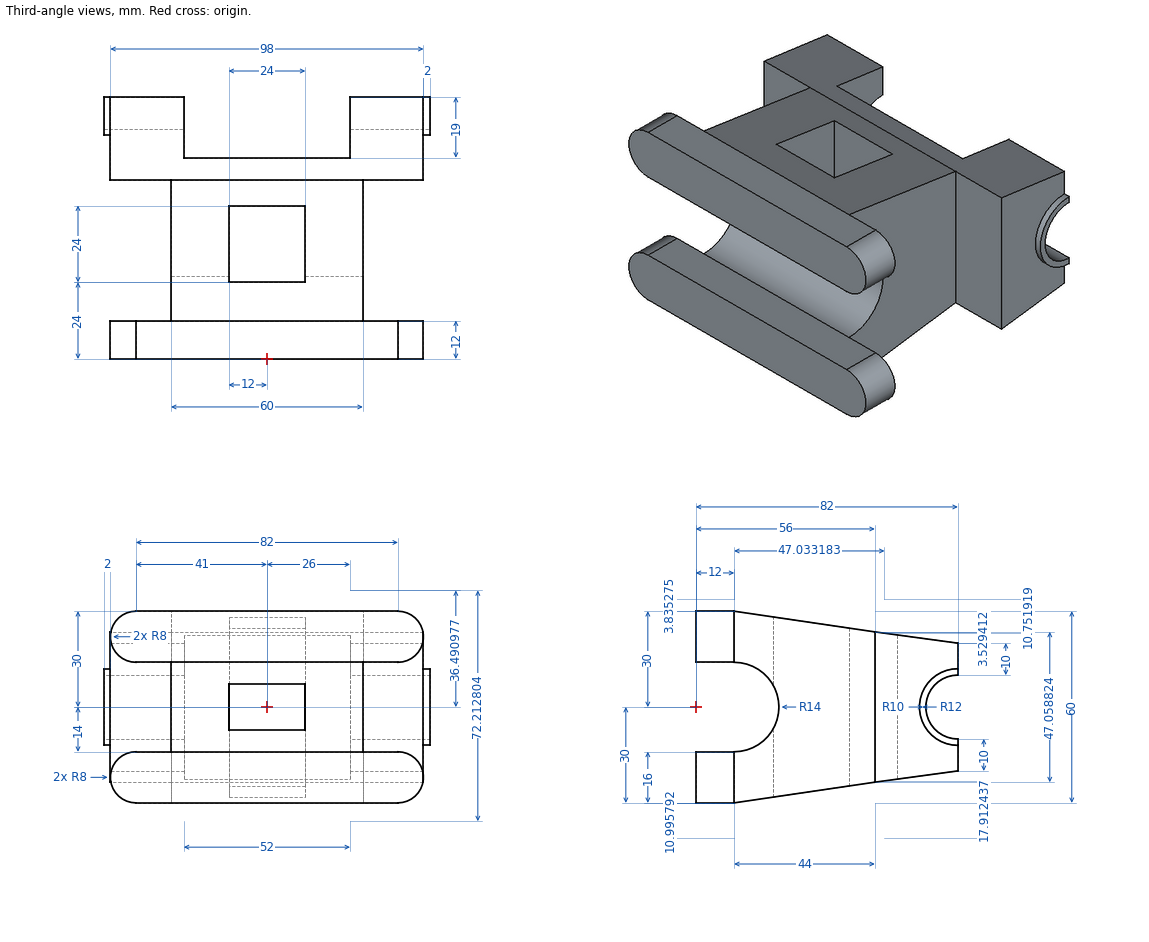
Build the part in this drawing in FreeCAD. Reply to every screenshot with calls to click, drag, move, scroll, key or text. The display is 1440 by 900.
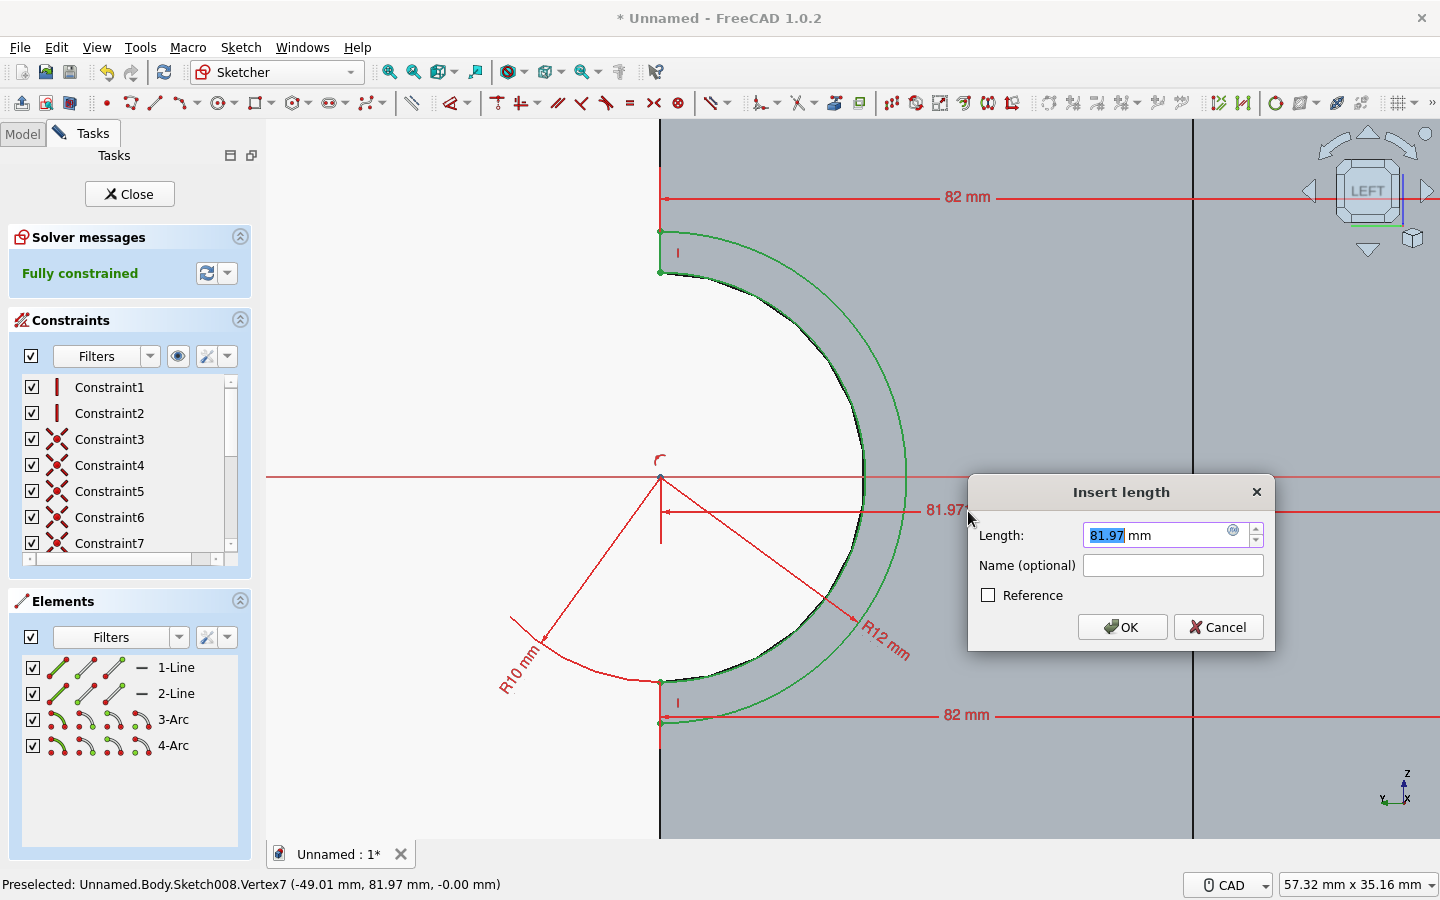
text(82)
key(Return)
key(Escape)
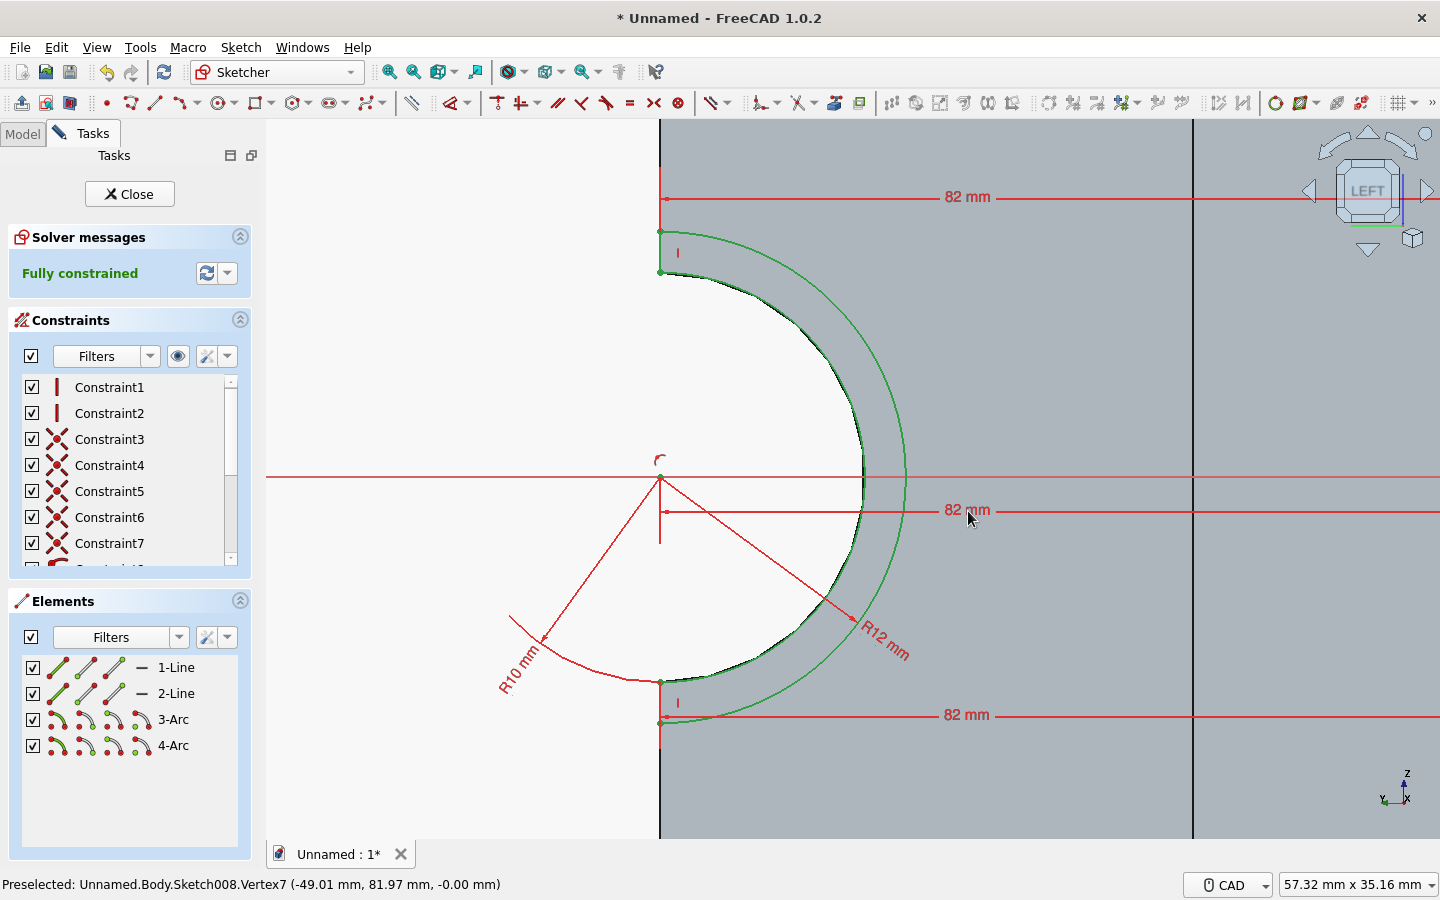
click(130, 194)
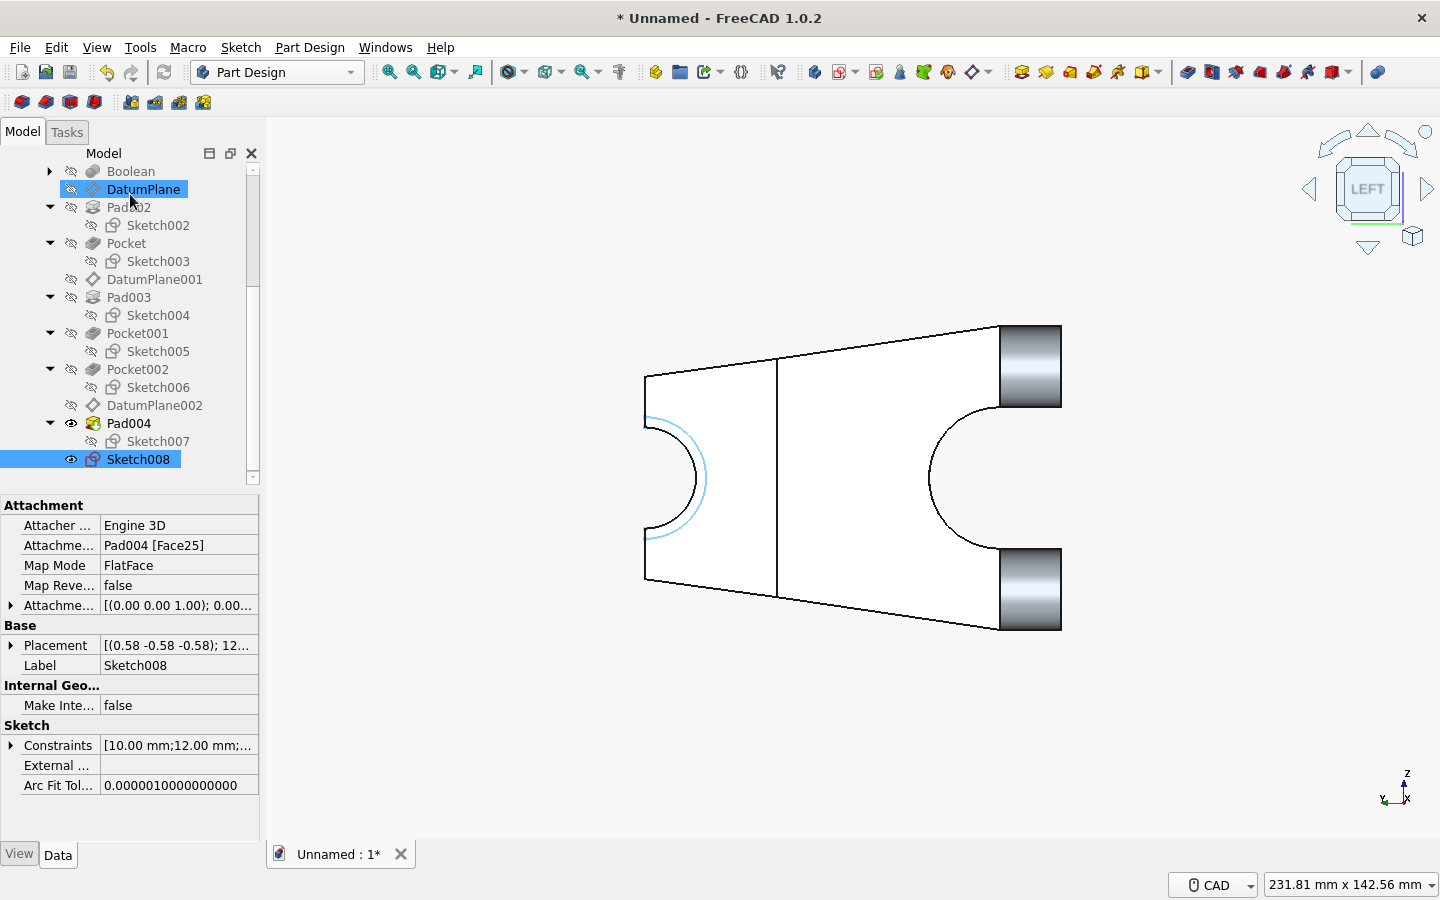
click(1022, 72)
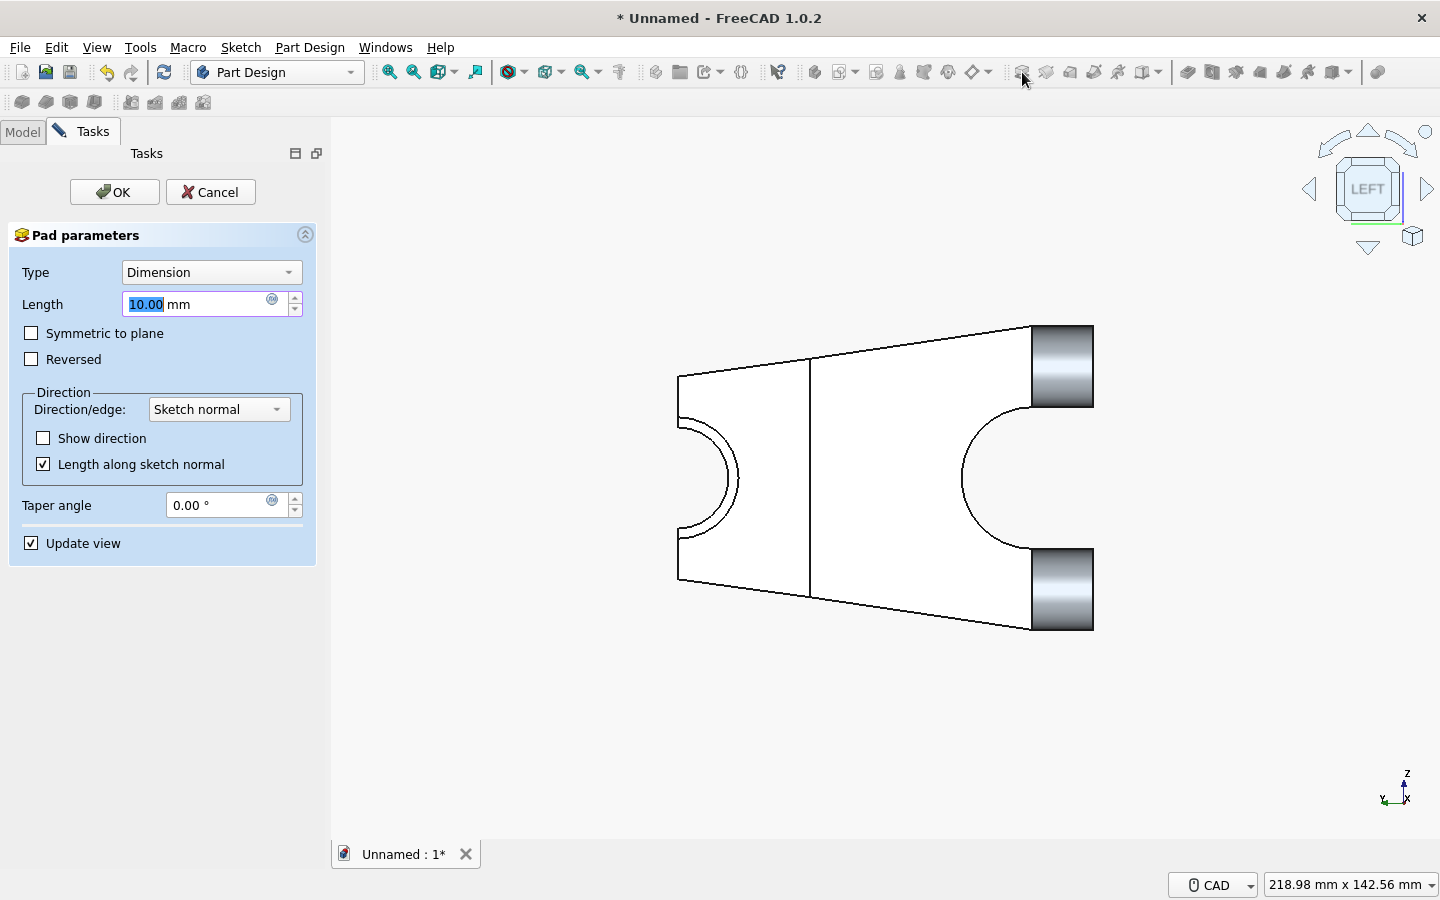
text(2)
key(Tab)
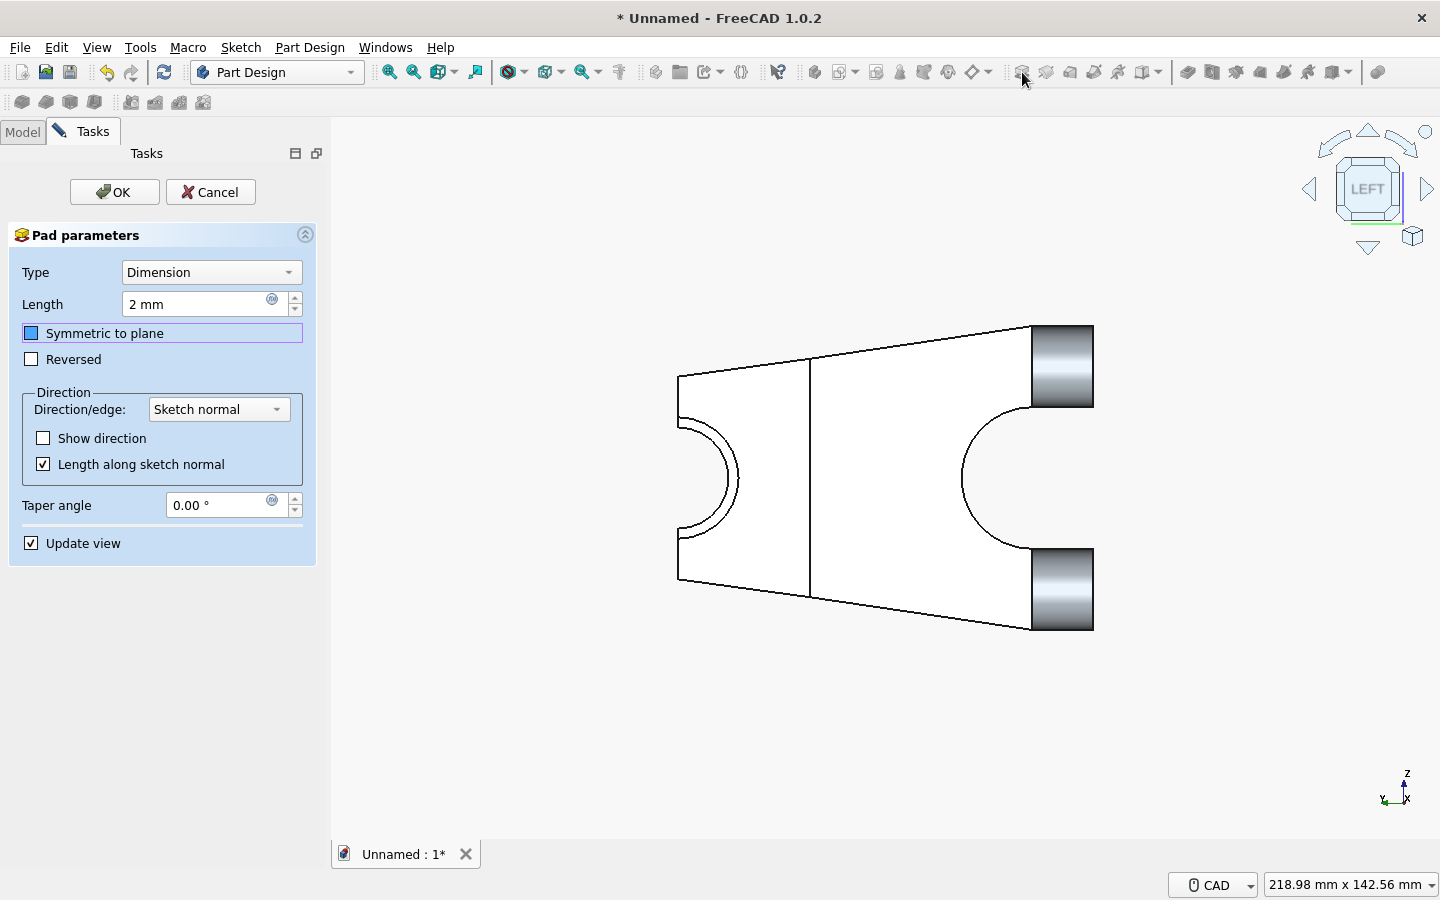
click(115, 192)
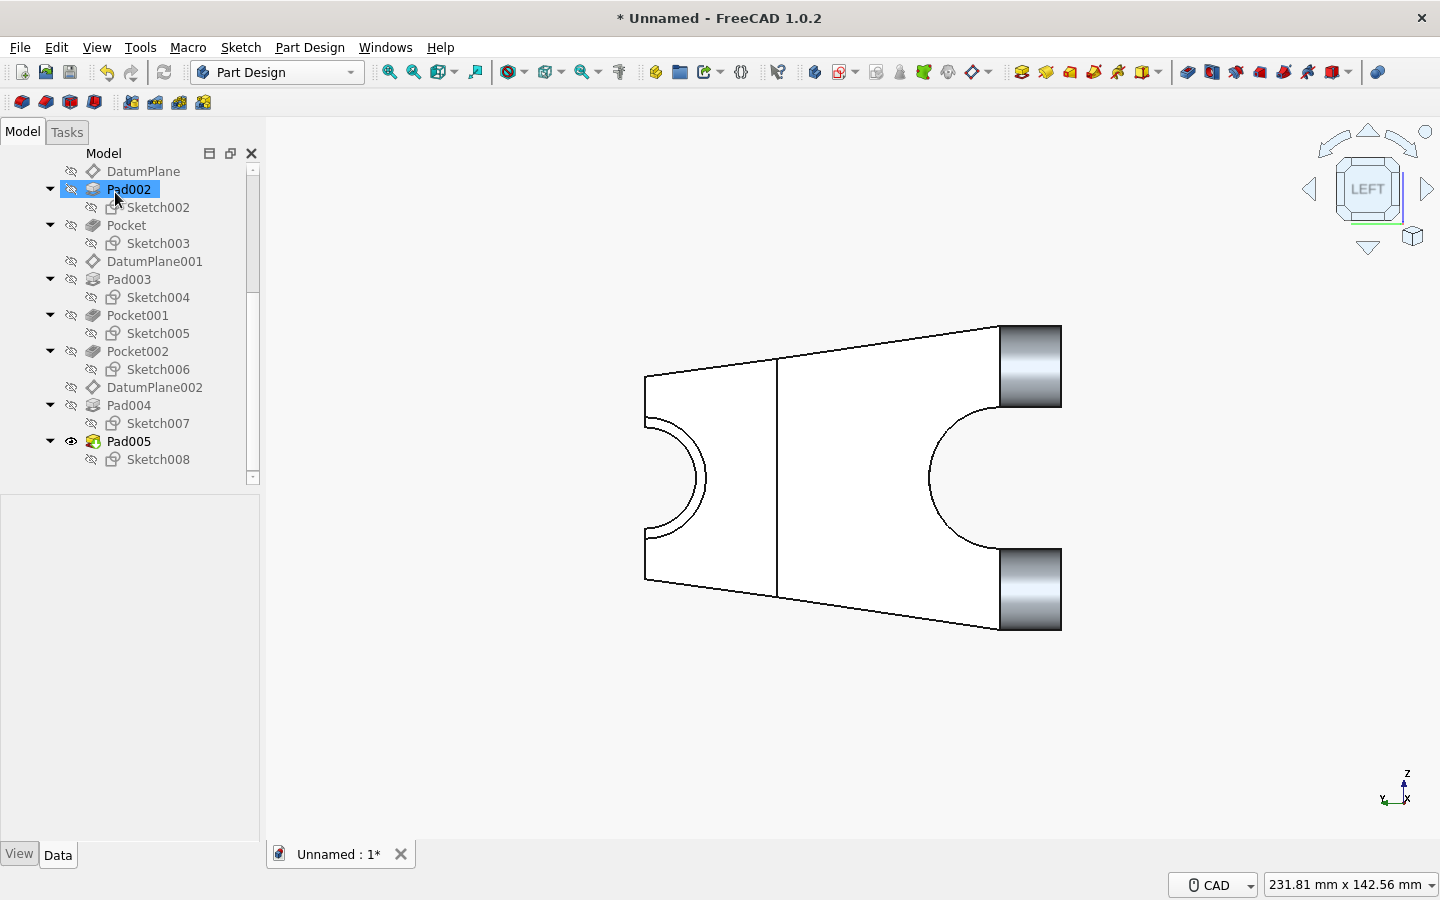
key(0)